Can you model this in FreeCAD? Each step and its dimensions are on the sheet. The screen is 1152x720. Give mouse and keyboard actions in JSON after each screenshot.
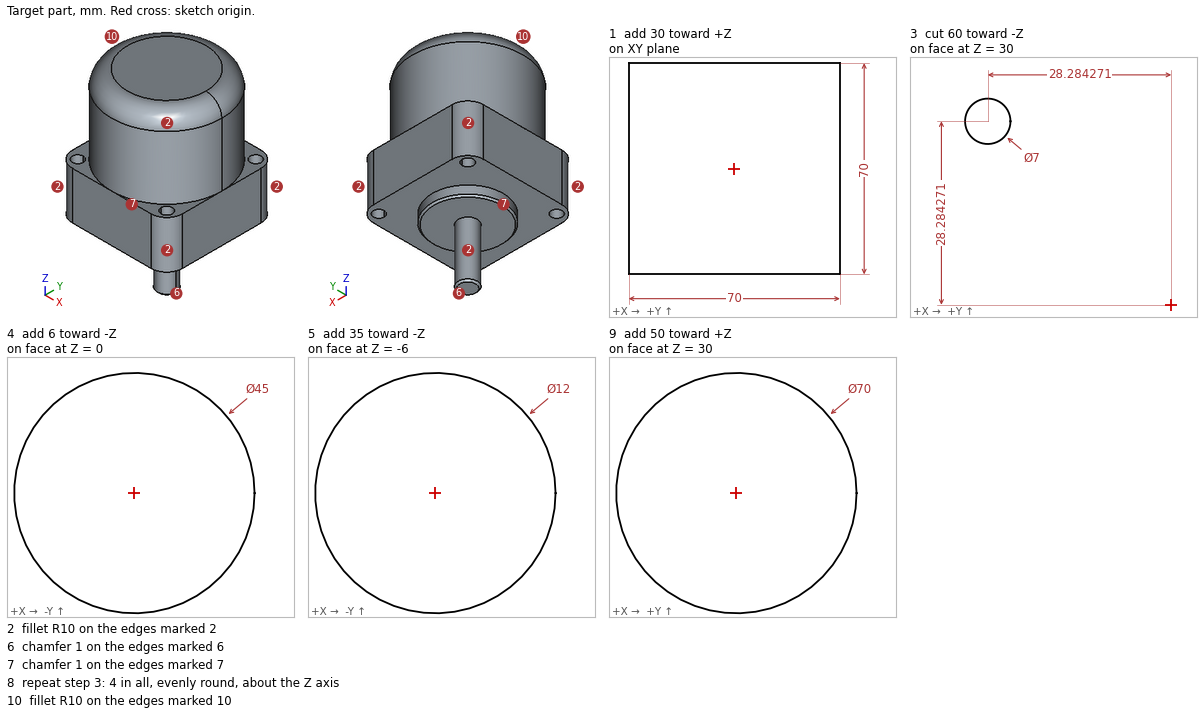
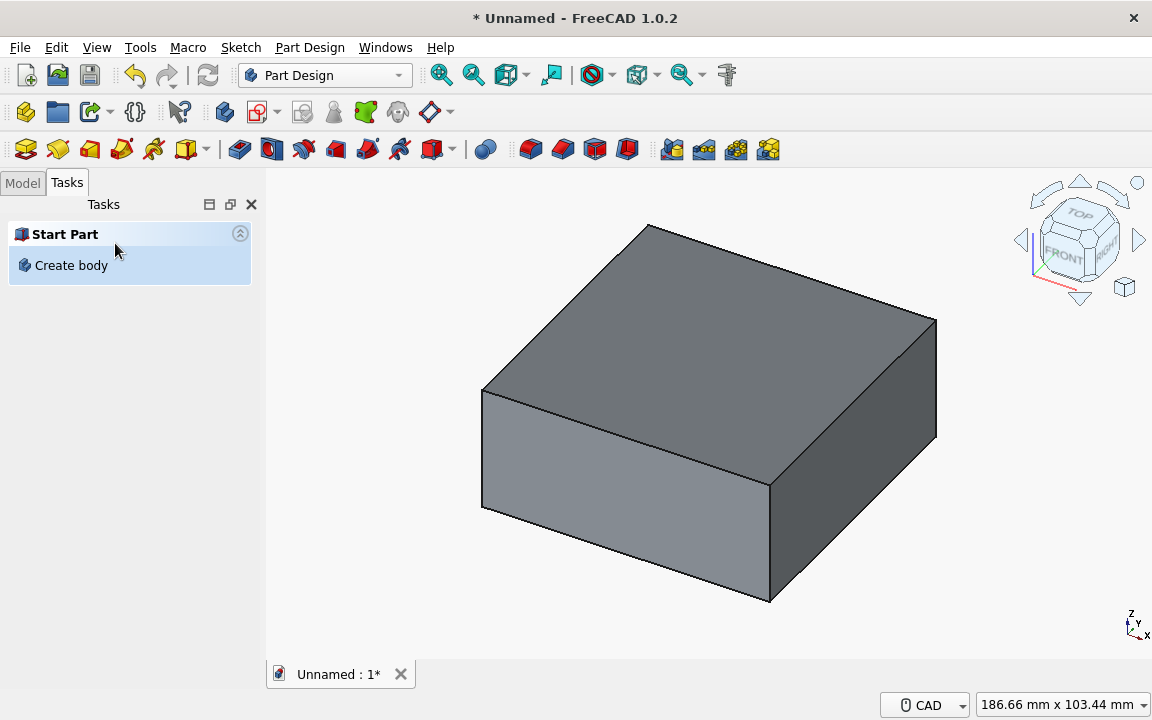
{"action": "left_click", "coordinate": [770, 543]}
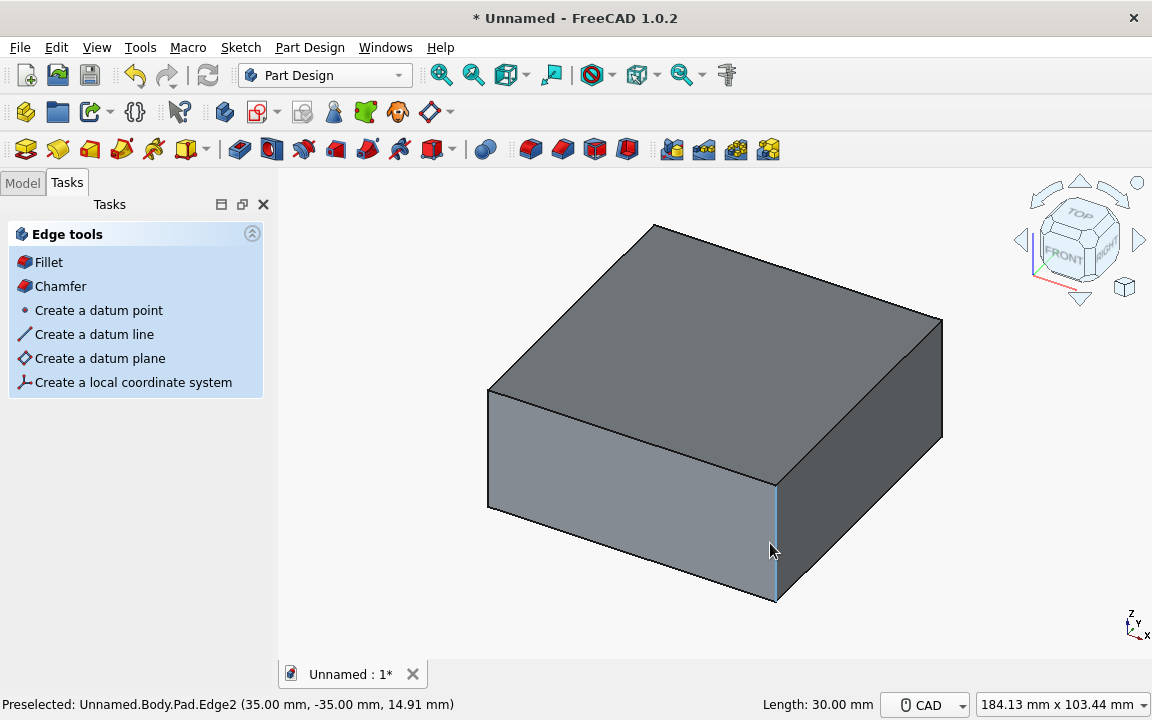
{"action": "key", "text": "0"}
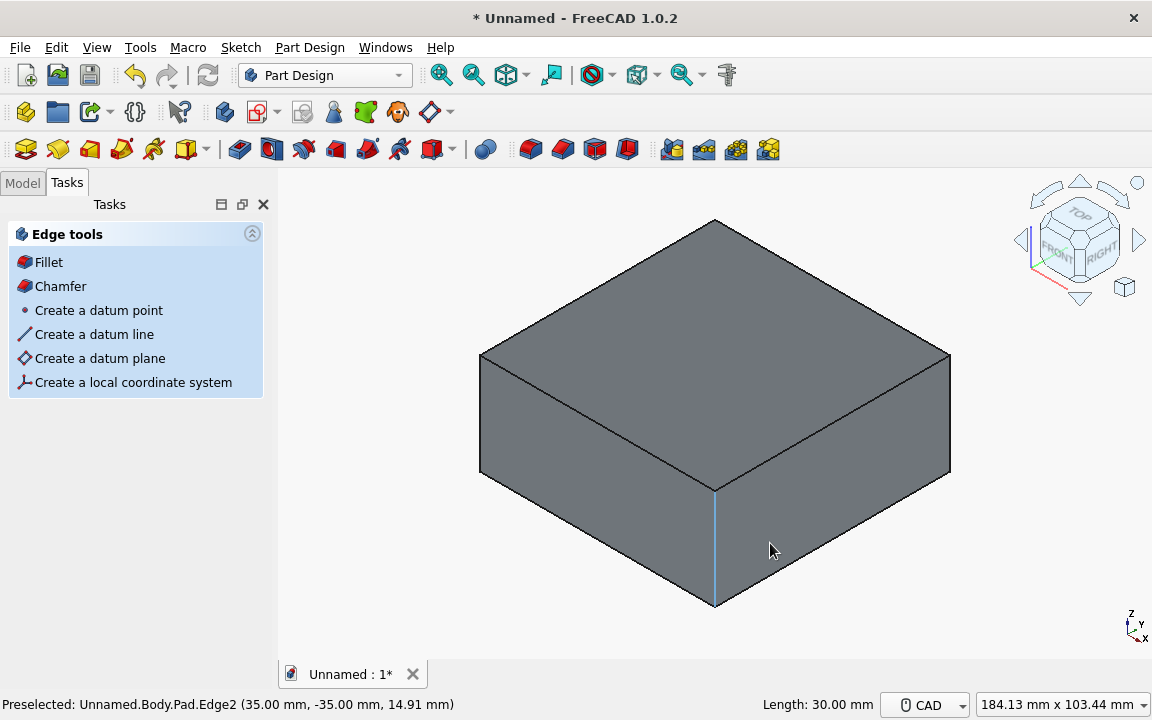
{"action": "key", "text": "2"}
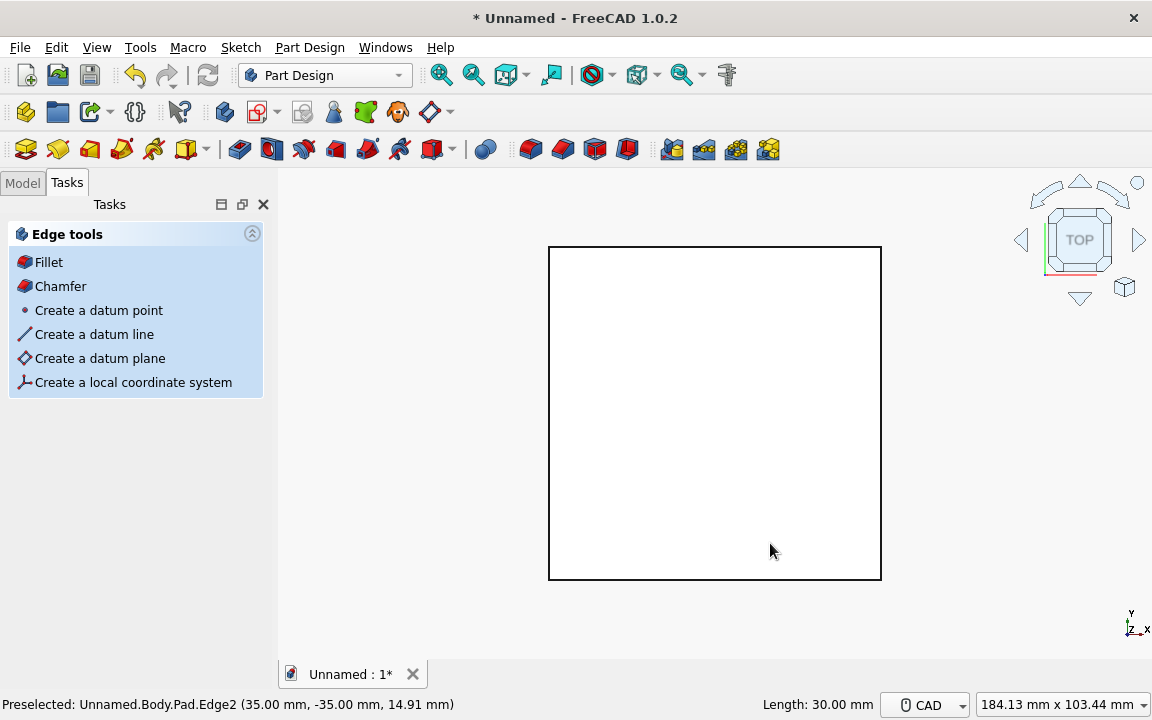
{"action": "key", "text": "1"}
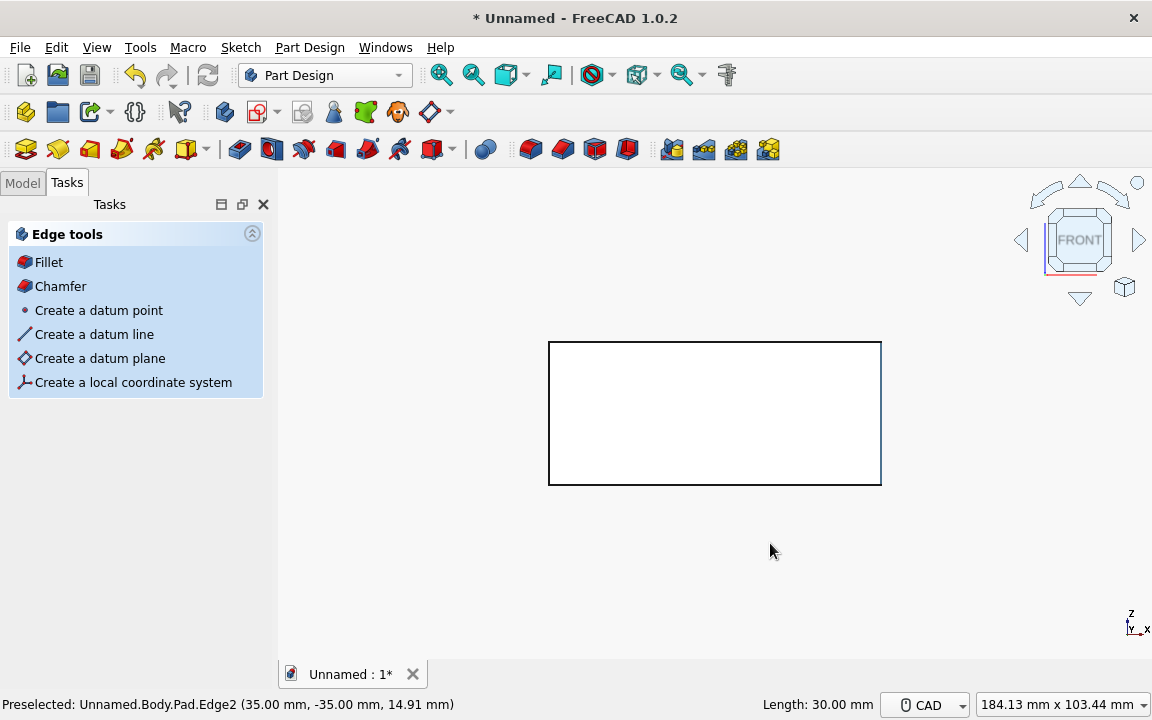
{"action": "key", "text": "v f"}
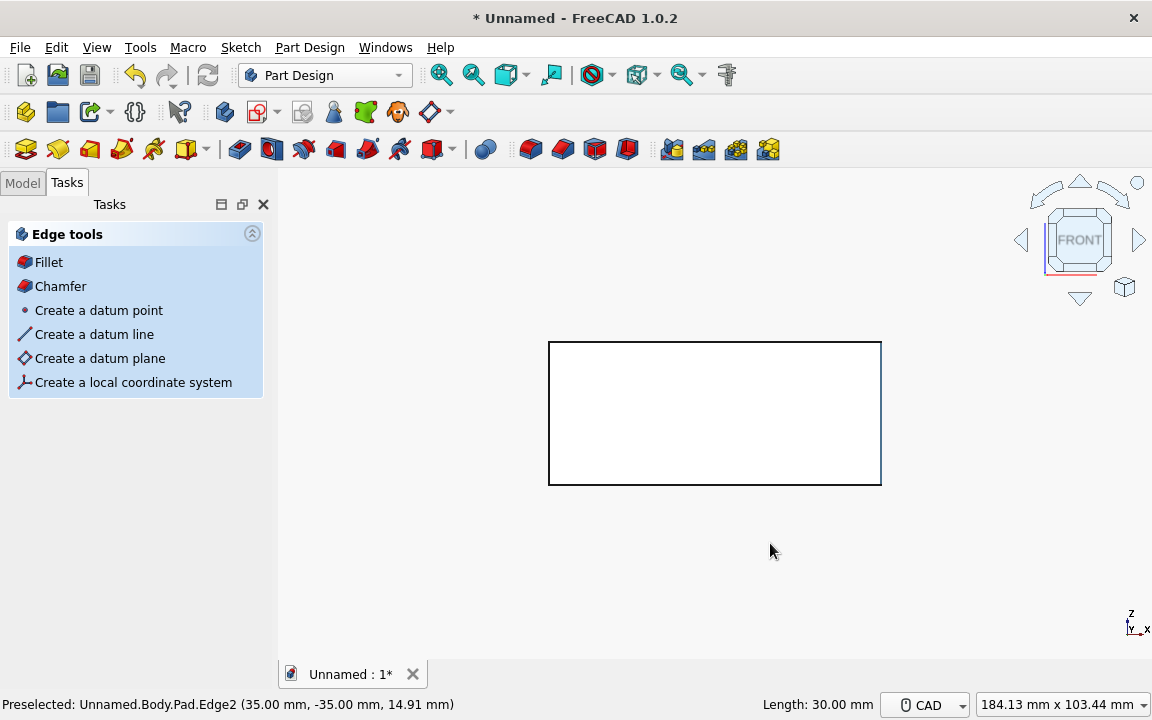
{"action": "left_click", "coordinate": [549, 413], "text": "ctrl"}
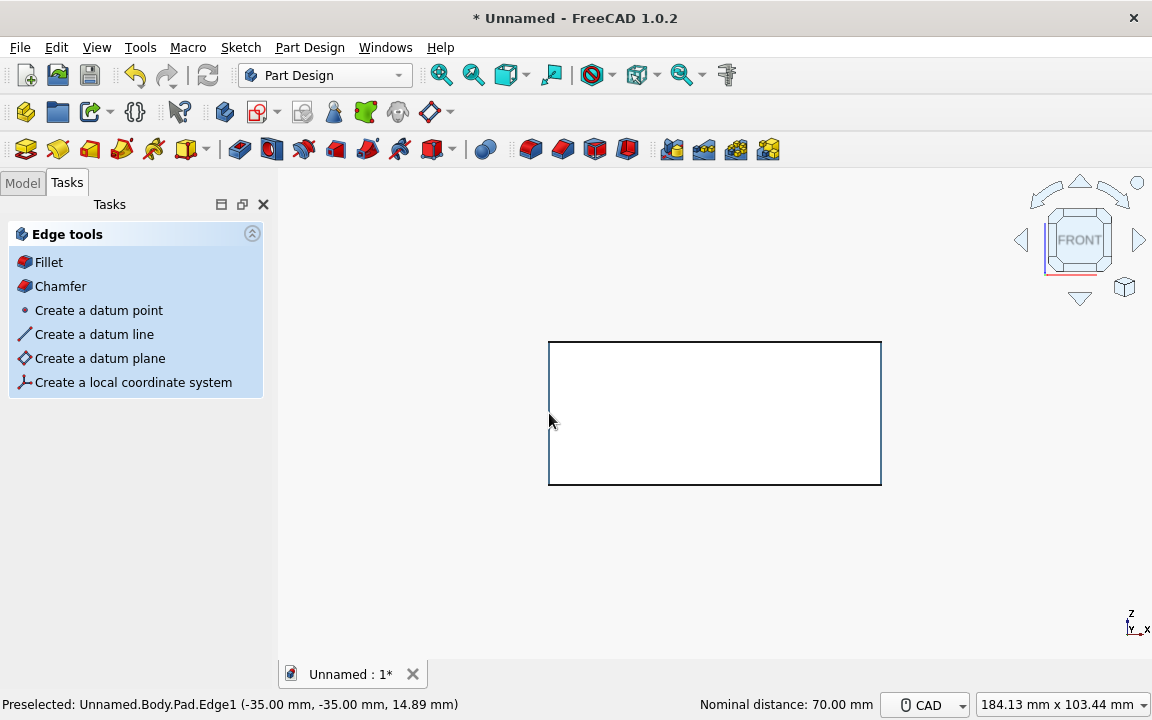
{"action": "key", "text": "3"}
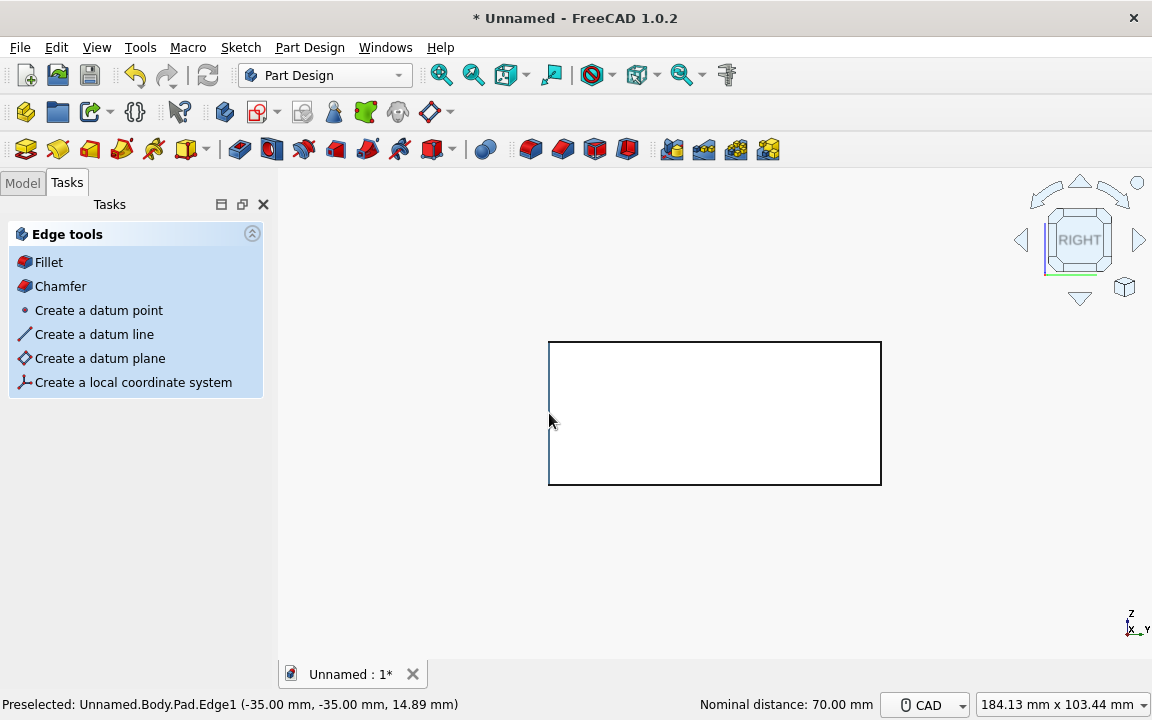
{"action": "left_click", "coordinate": [442, 76]}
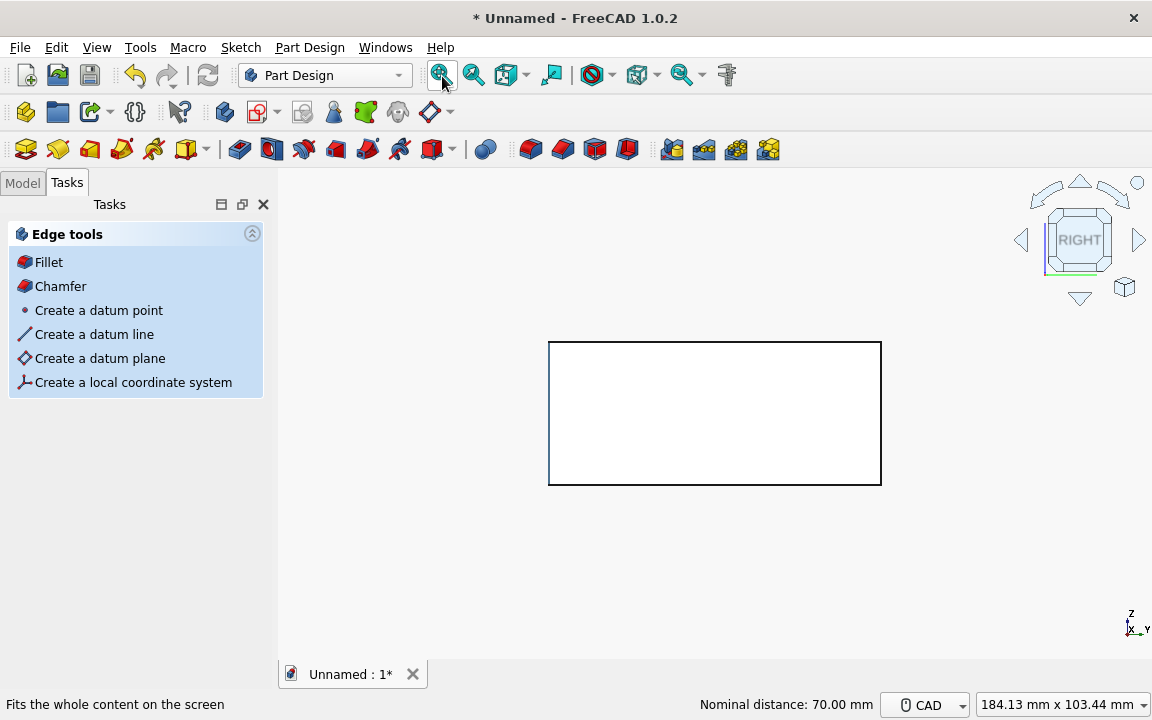
{"action": "left_click", "coordinate": [881, 412], "text": "ctrl"}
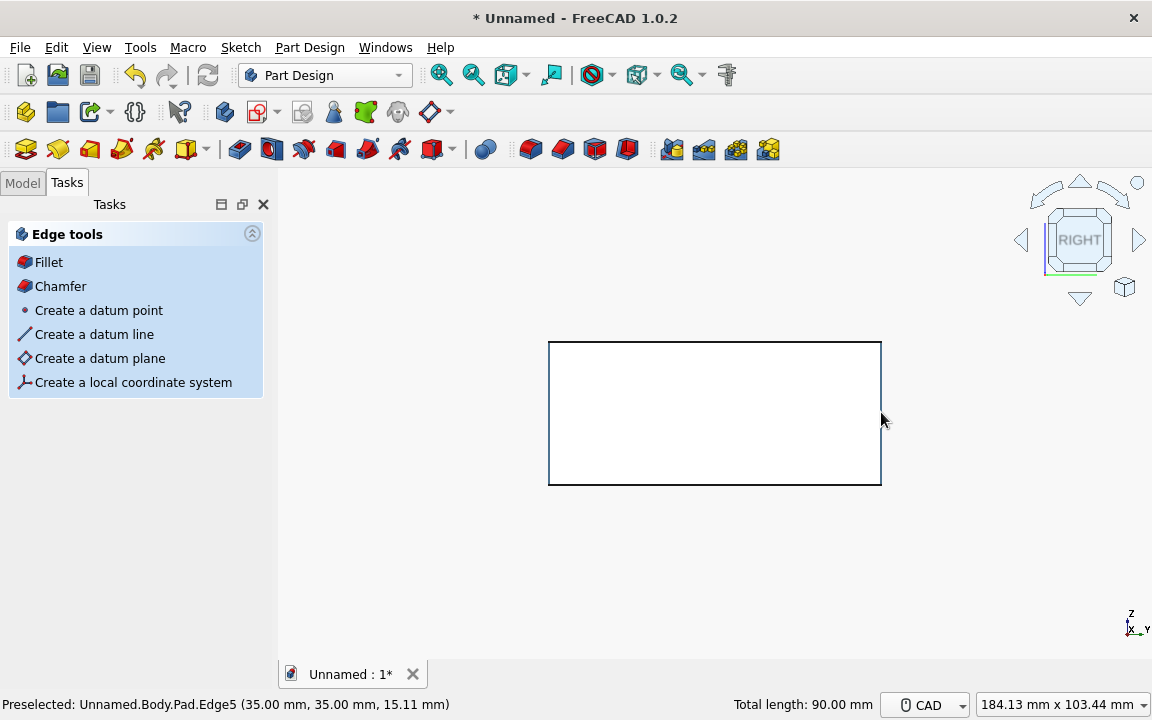
{"action": "key", "text": "5"}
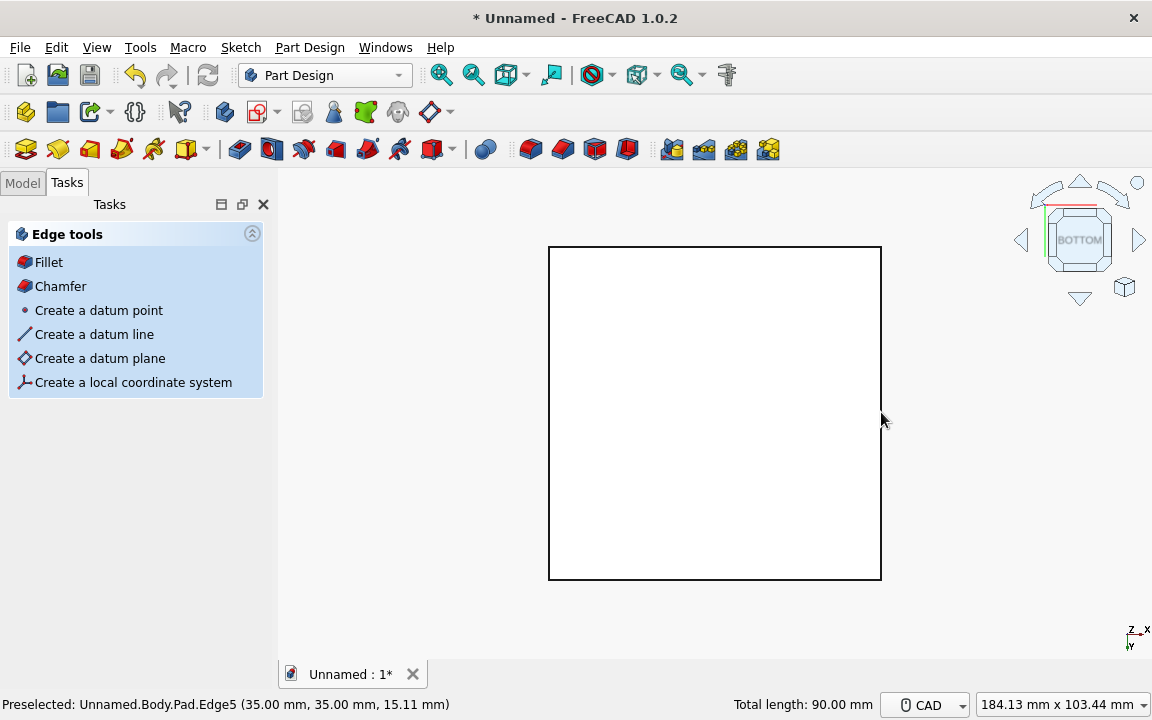
{"action": "key", "text": "4"}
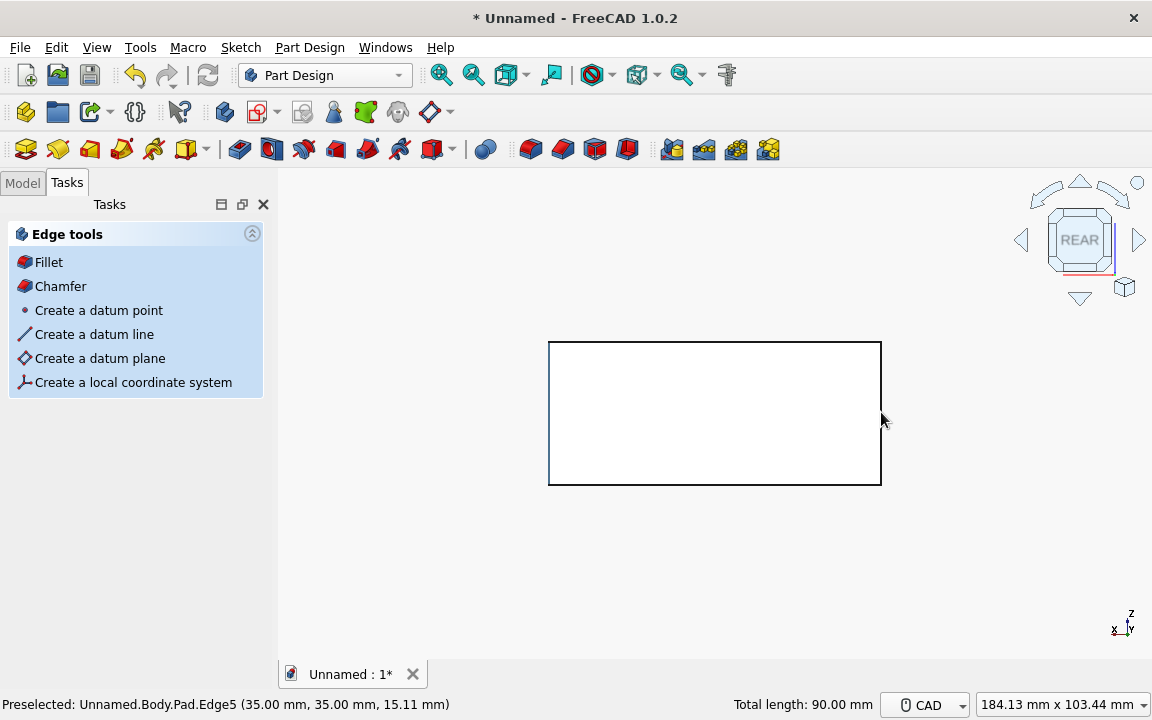
{"action": "key", "text": "v f"}